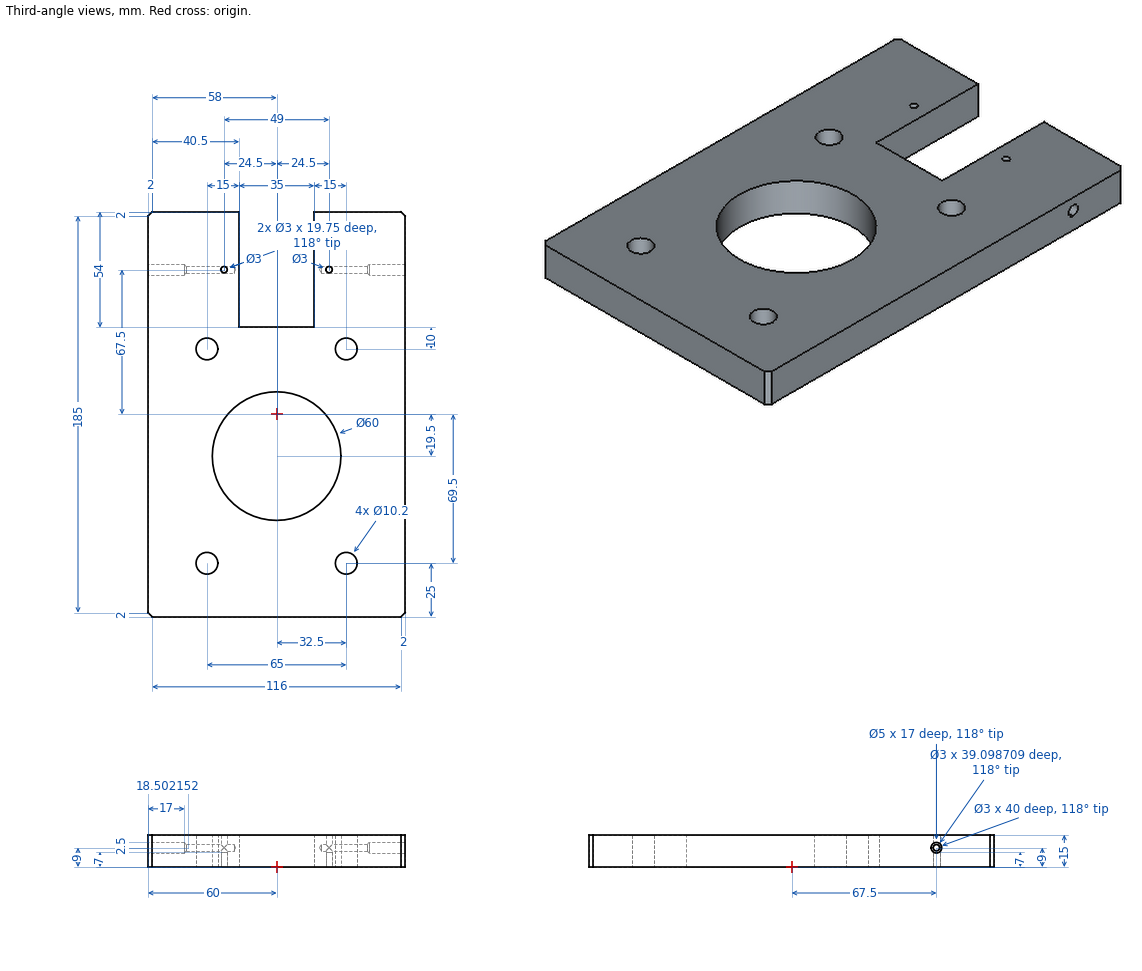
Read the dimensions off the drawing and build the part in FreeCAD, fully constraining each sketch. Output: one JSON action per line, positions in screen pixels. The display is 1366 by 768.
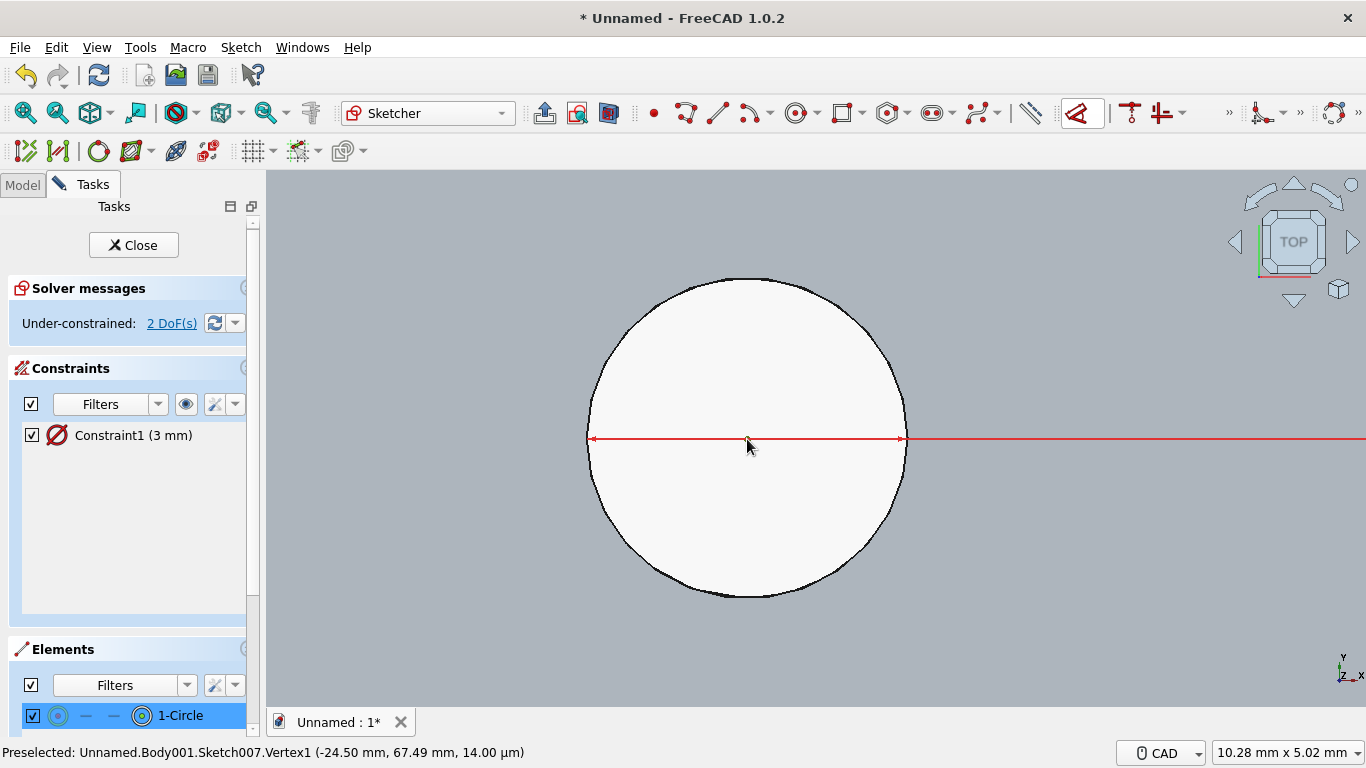
{"action": "key", "text": "l"}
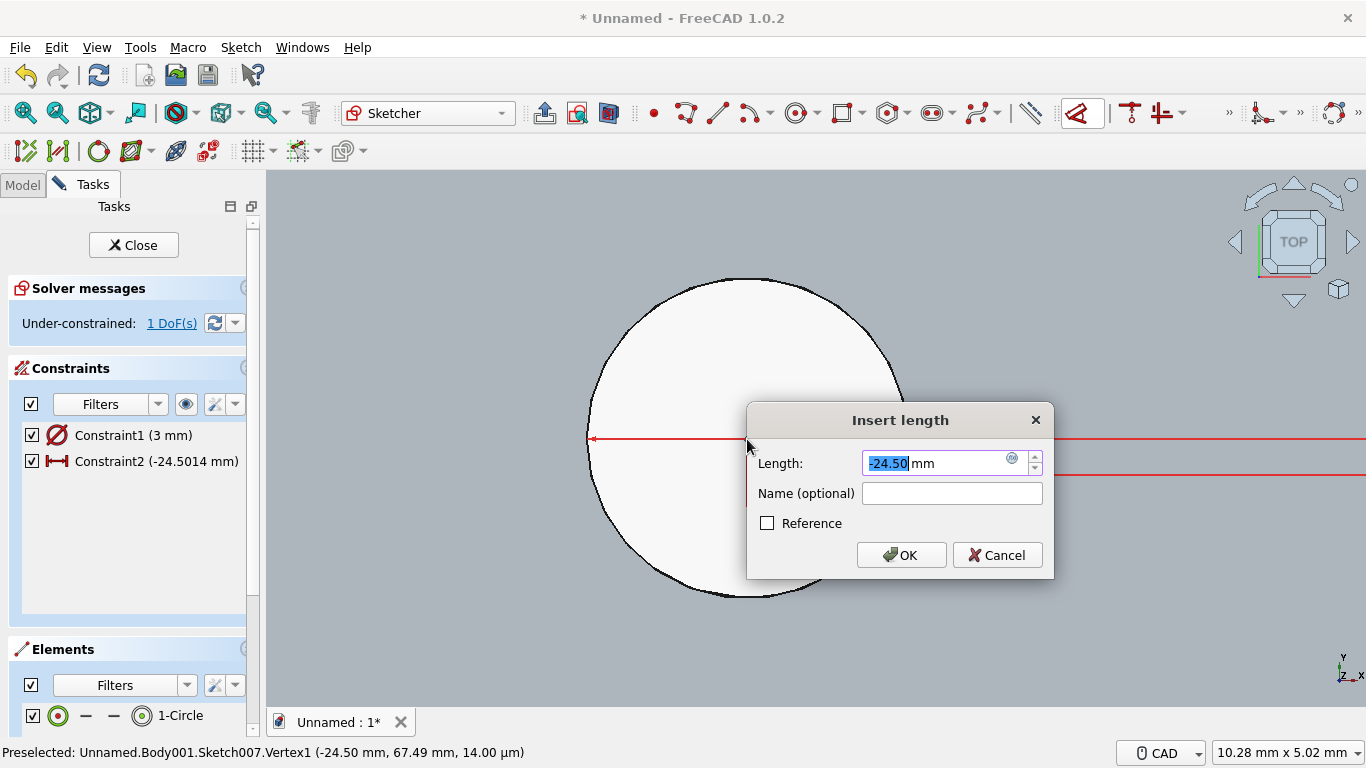
{"action": "type", "text": "-24.5"}
{"action": "key", "text": "Return"}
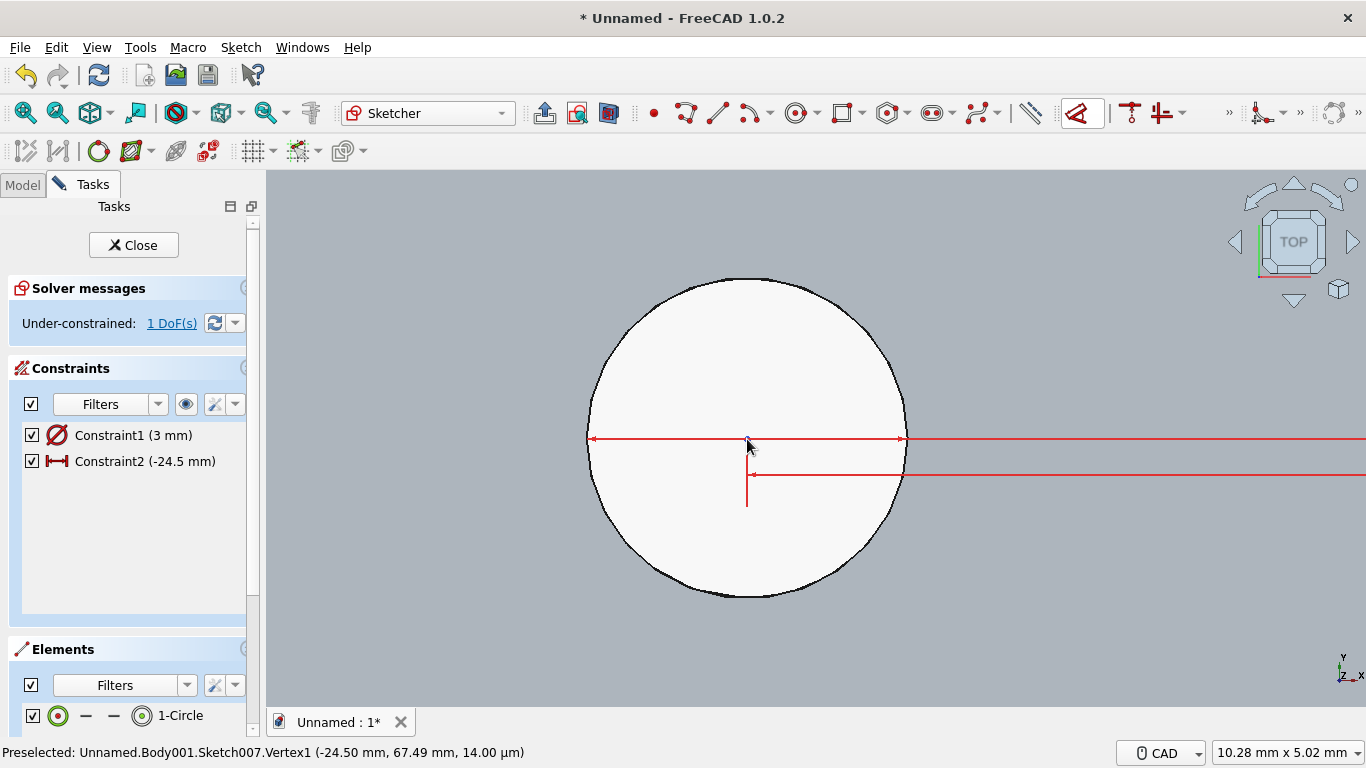
{"action": "left_click", "coordinate": [747, 439]}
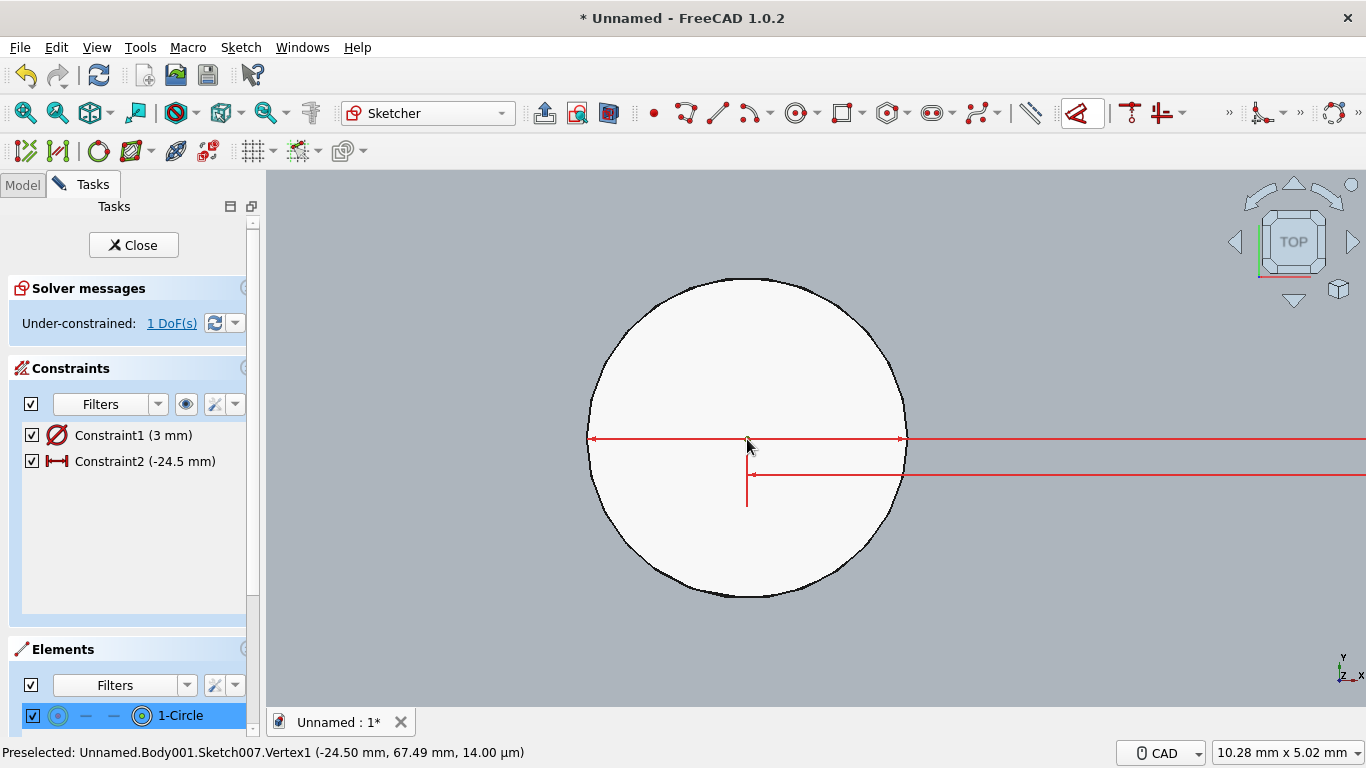
{"action": "left_click", "coordinate": [1098, 114]}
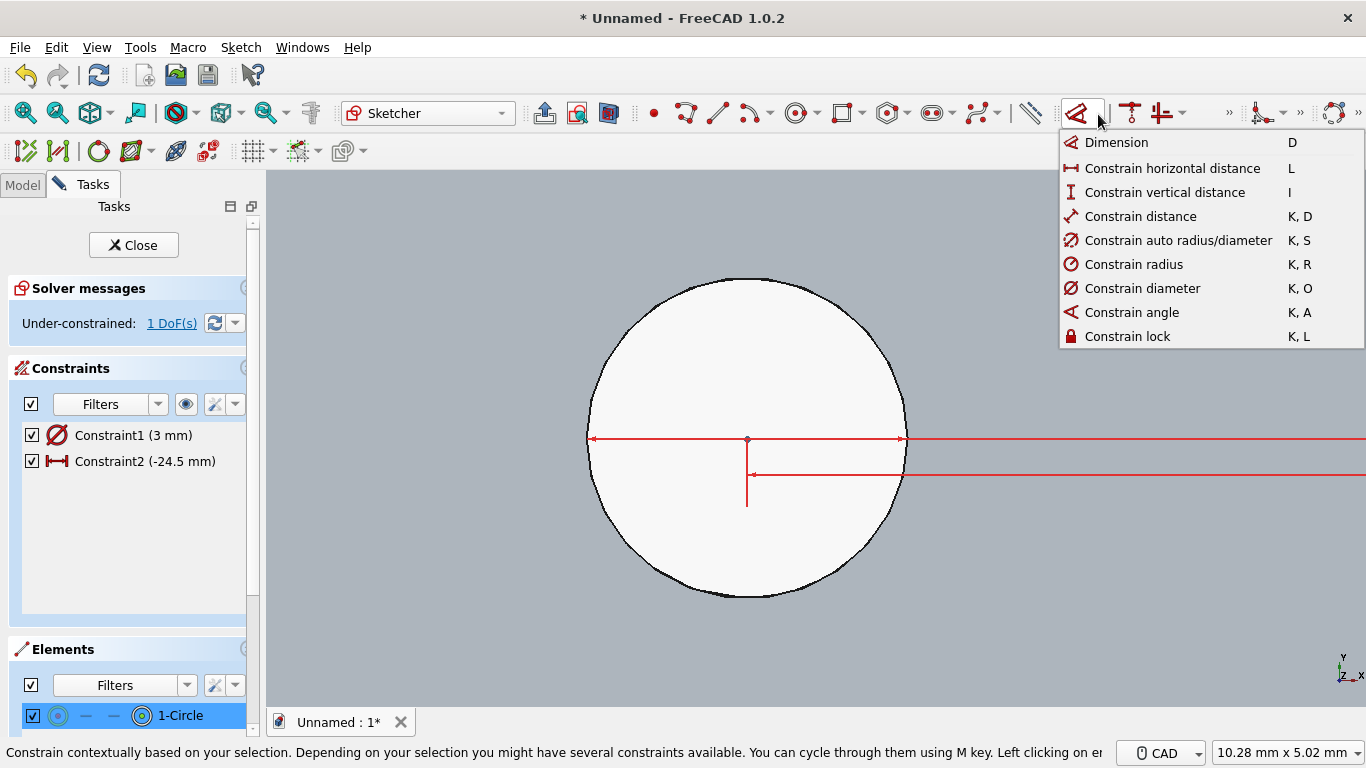
{"action": "left_click", "coordinate": [1212, 192]}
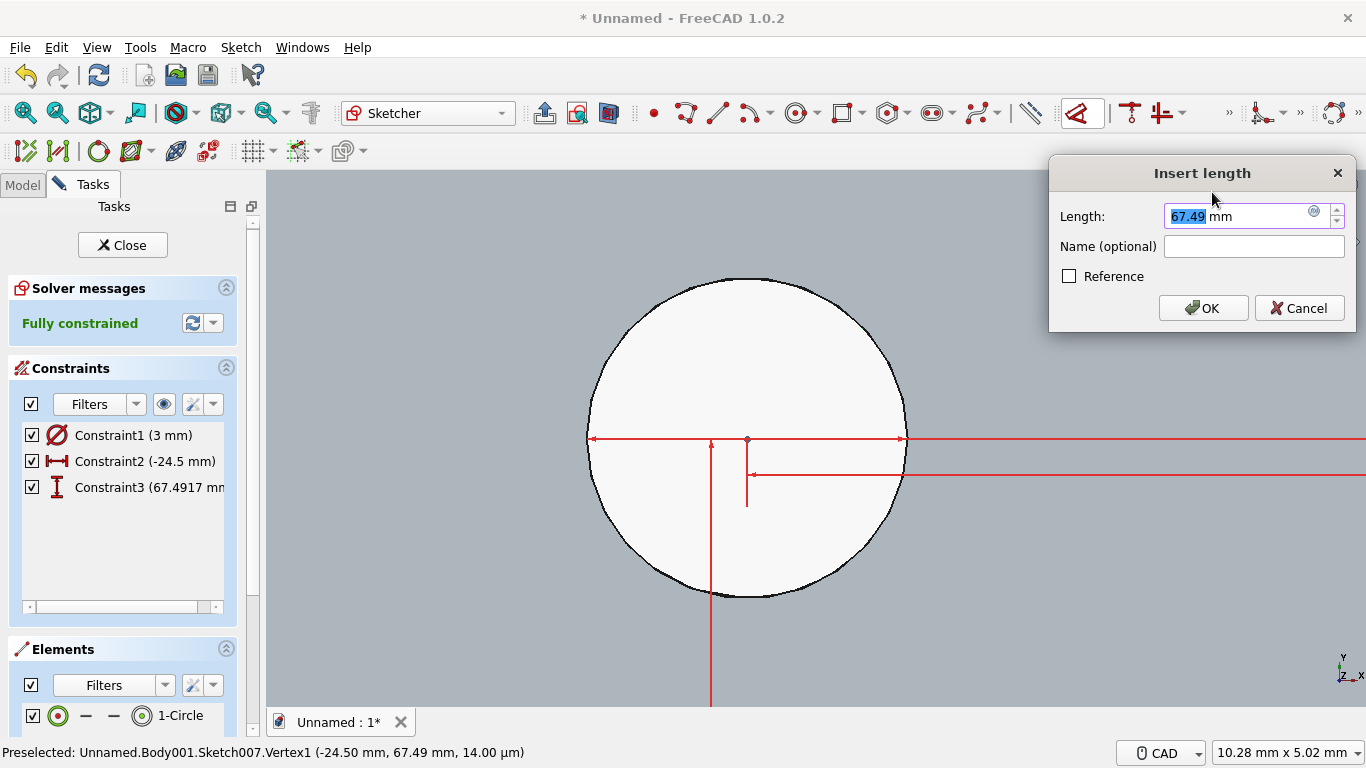
{"action": "type", "text": "67.5"}
{"action": "key", "text": "Return"}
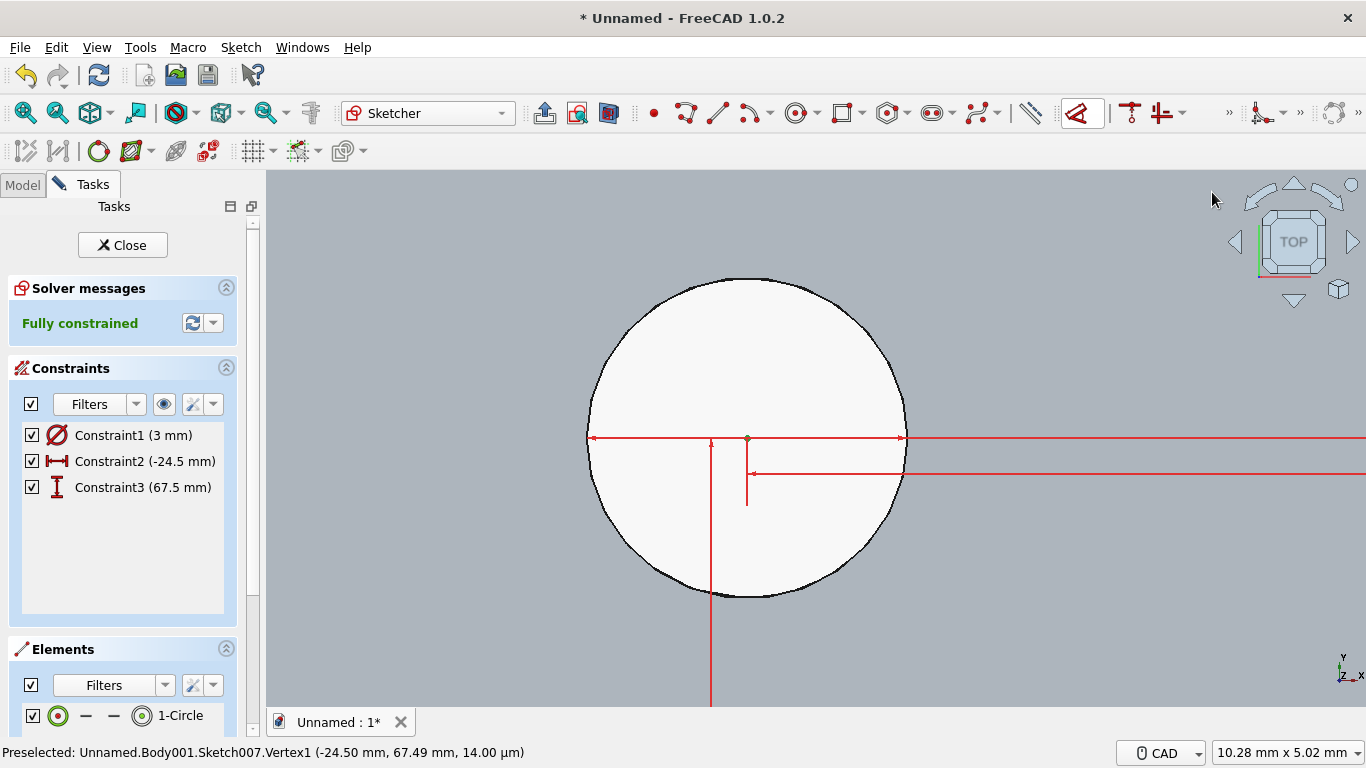
{"action": "left_click", "coordinate": [123, 245]}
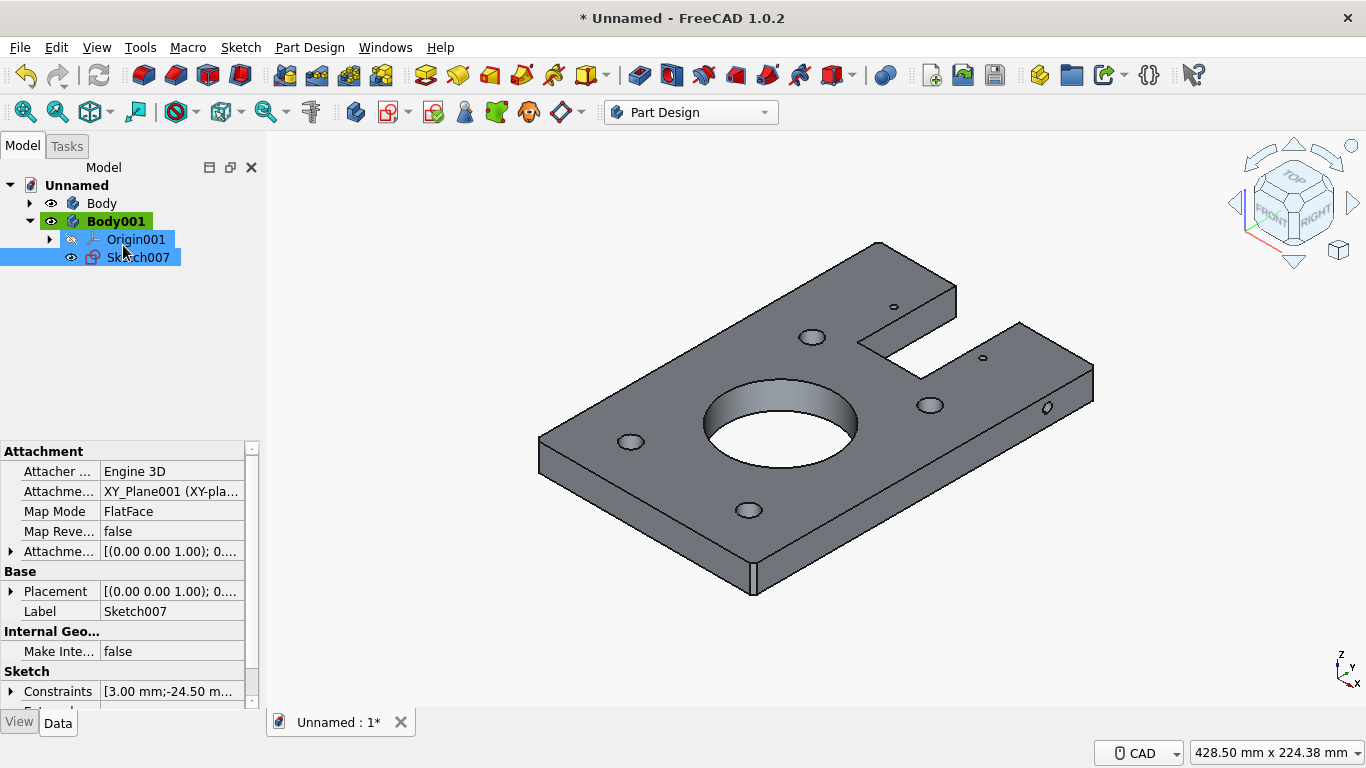
{"action": "left_click", "coordinate": [426, 76]}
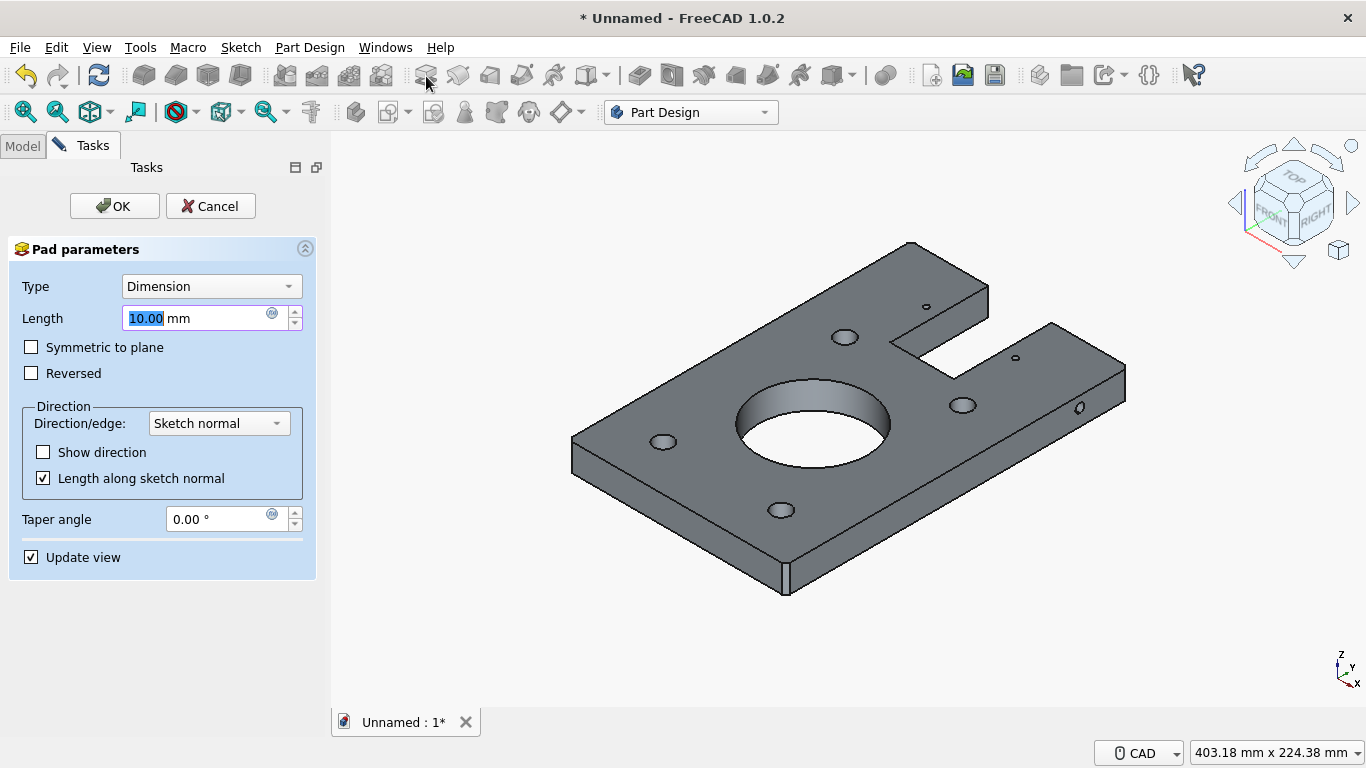
{"action": "type", "text": "7"}
{"action": "key", "text": "Tab"}